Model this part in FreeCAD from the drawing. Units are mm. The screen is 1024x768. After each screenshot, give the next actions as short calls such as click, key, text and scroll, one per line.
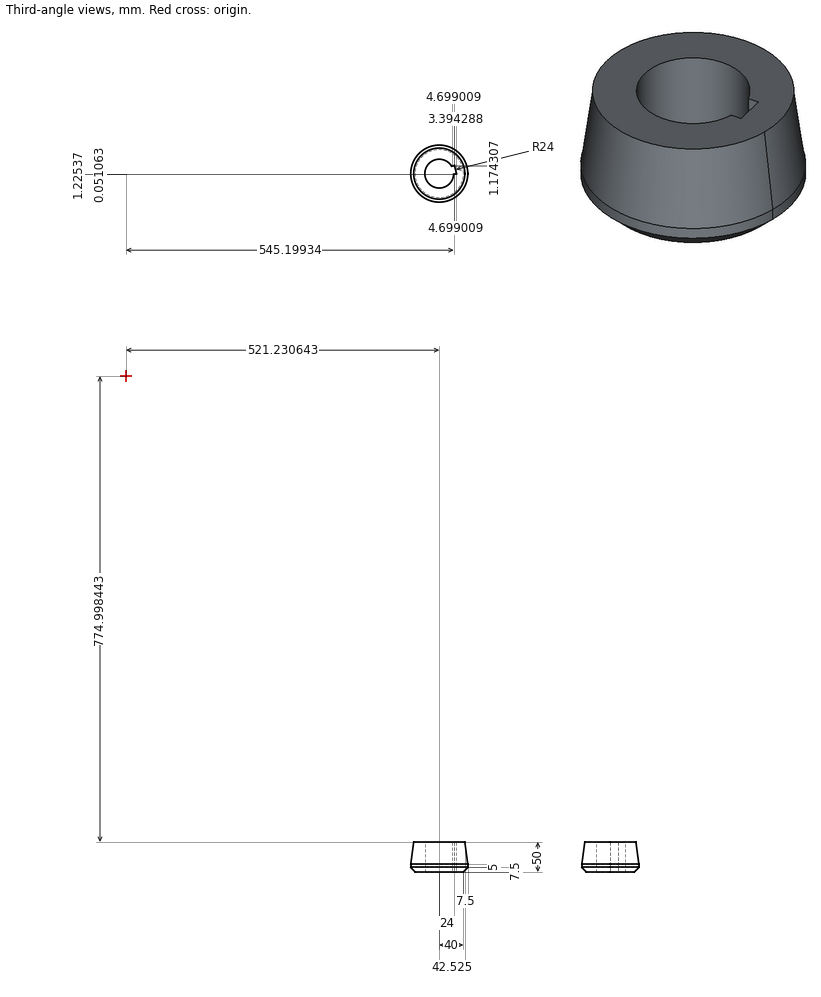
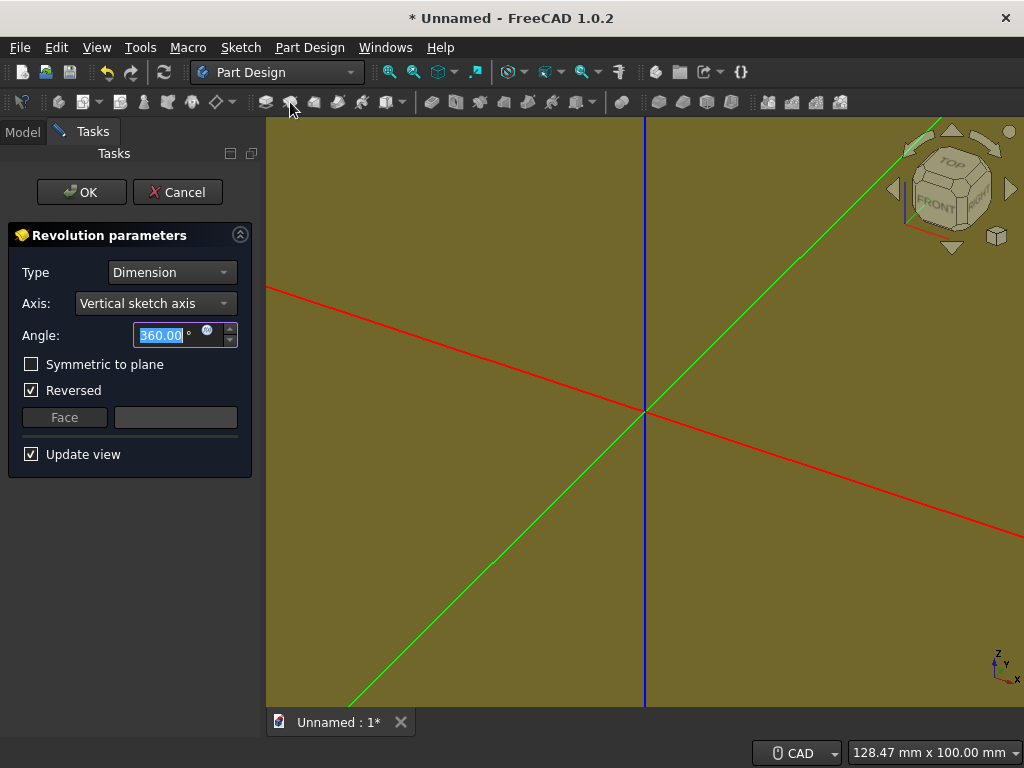
click(156, 304)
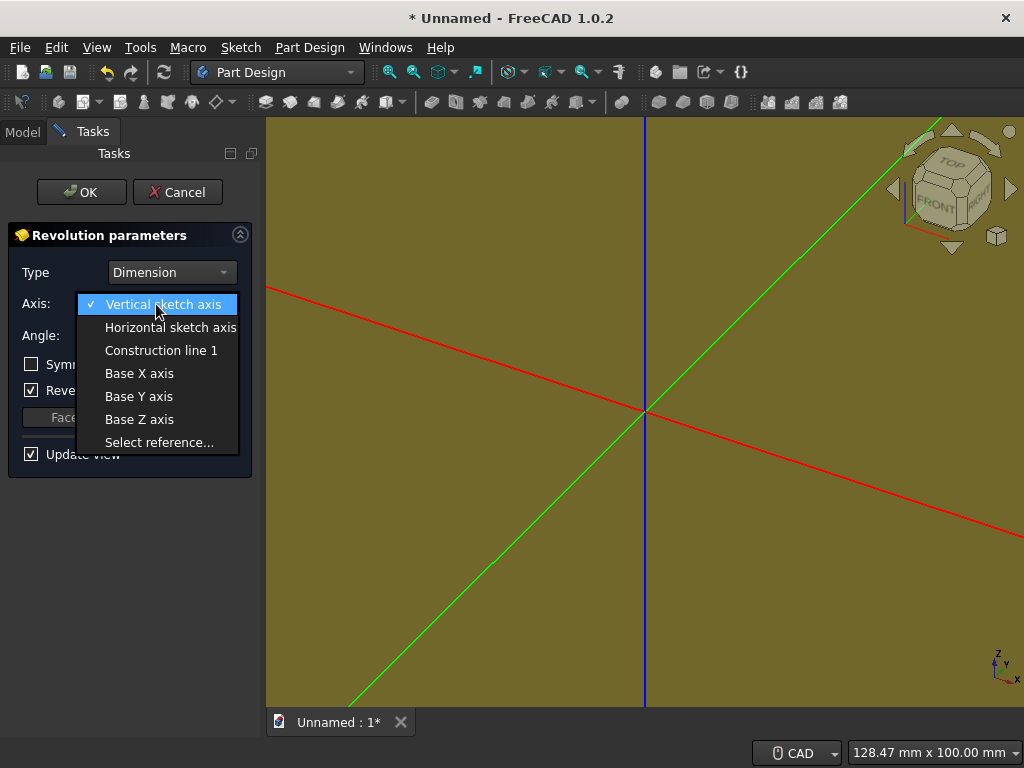
click(156, 350)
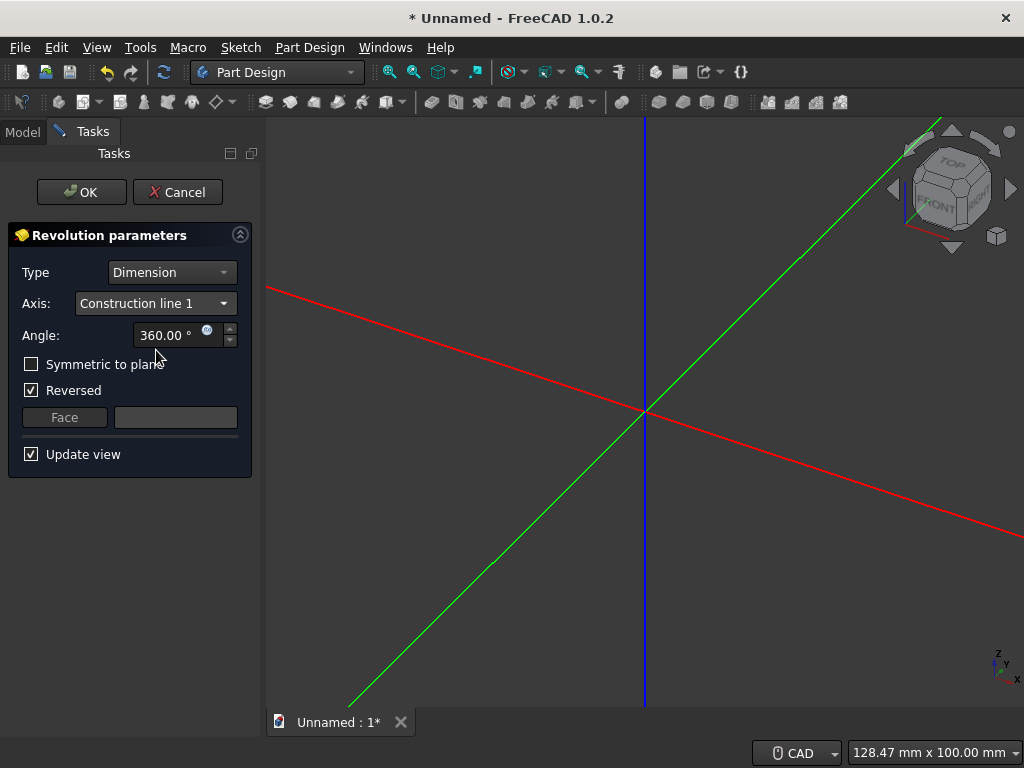
click(82, 192)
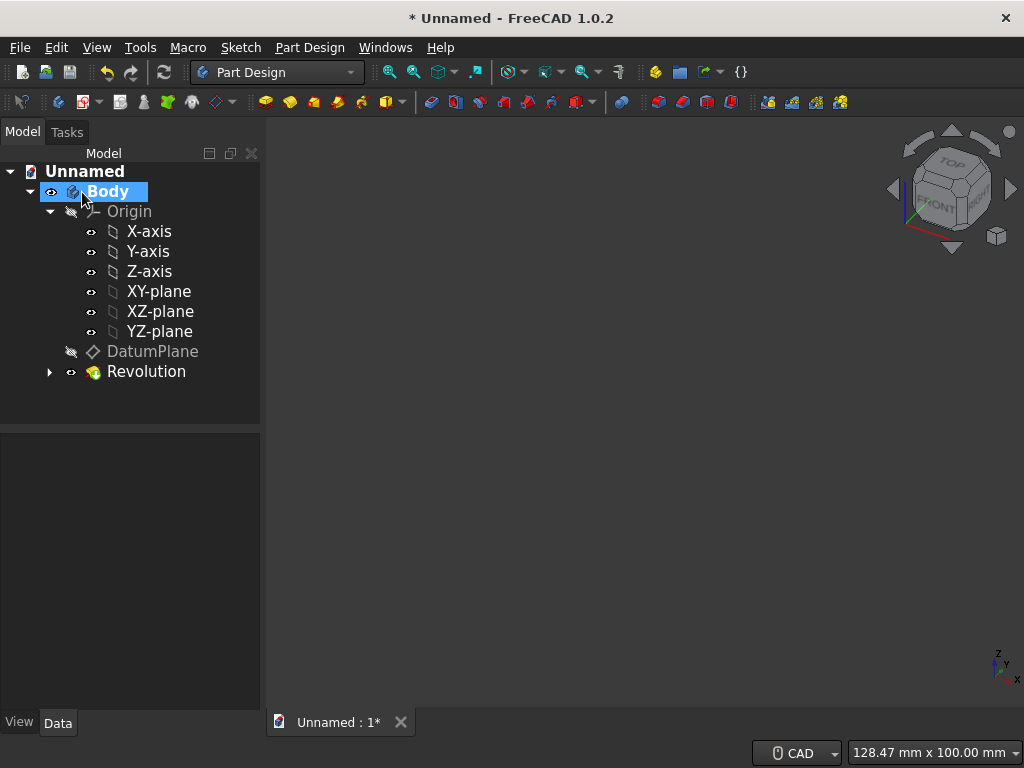
click(390, 72)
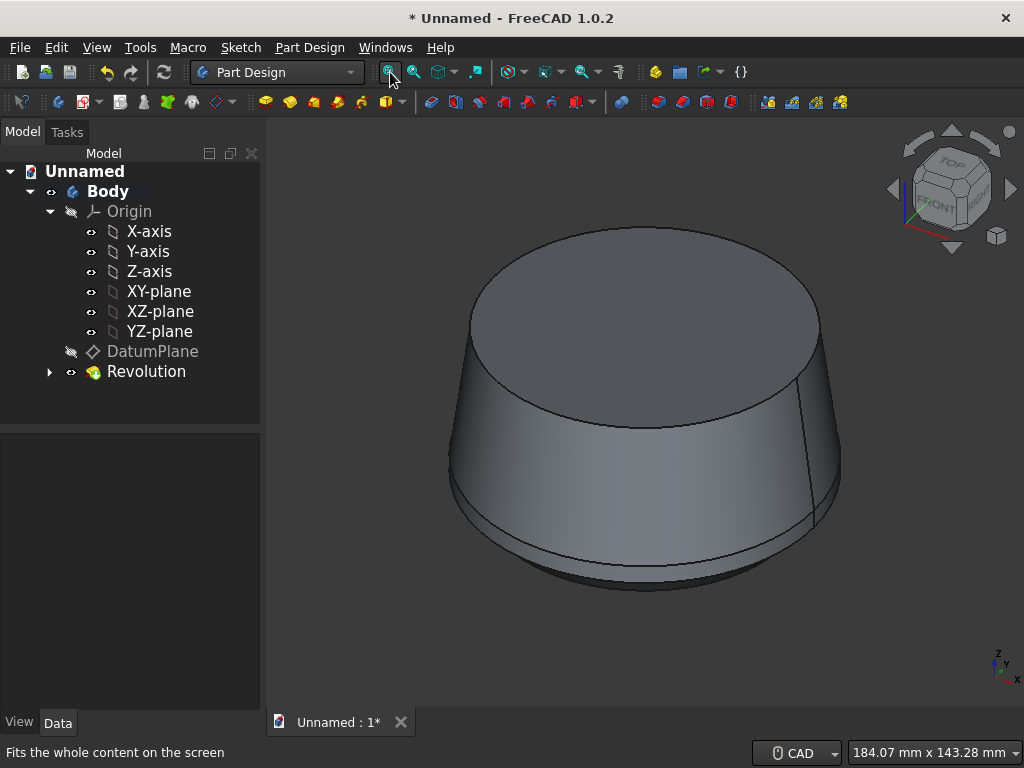
click(645, 327)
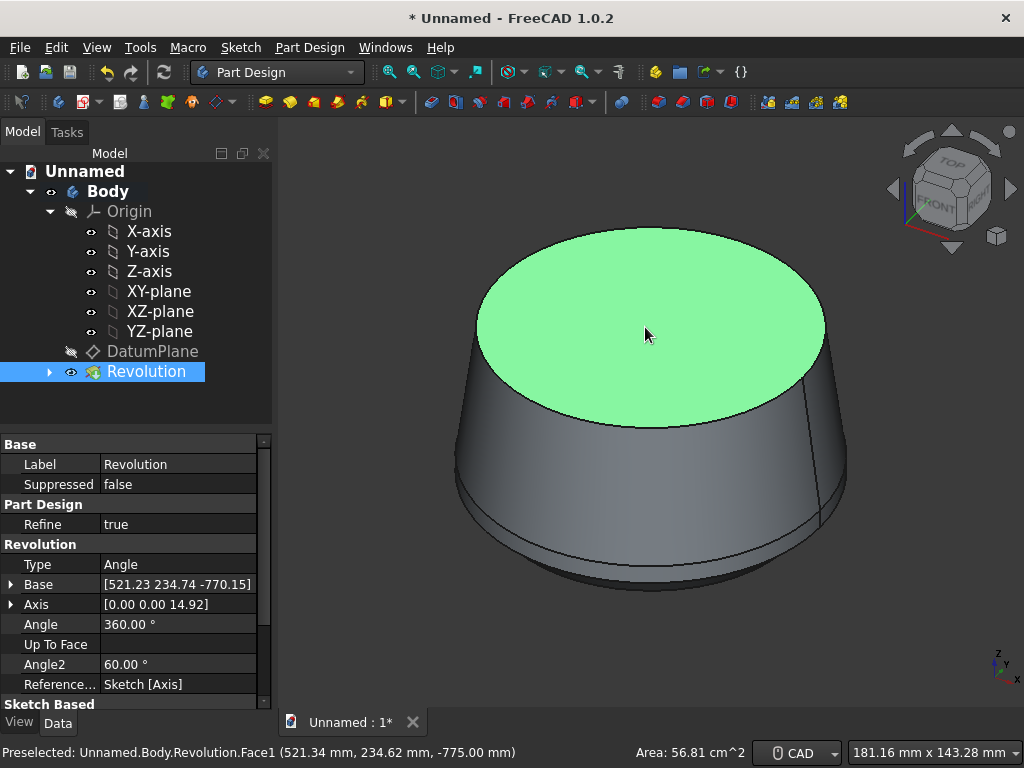
click(84, 102)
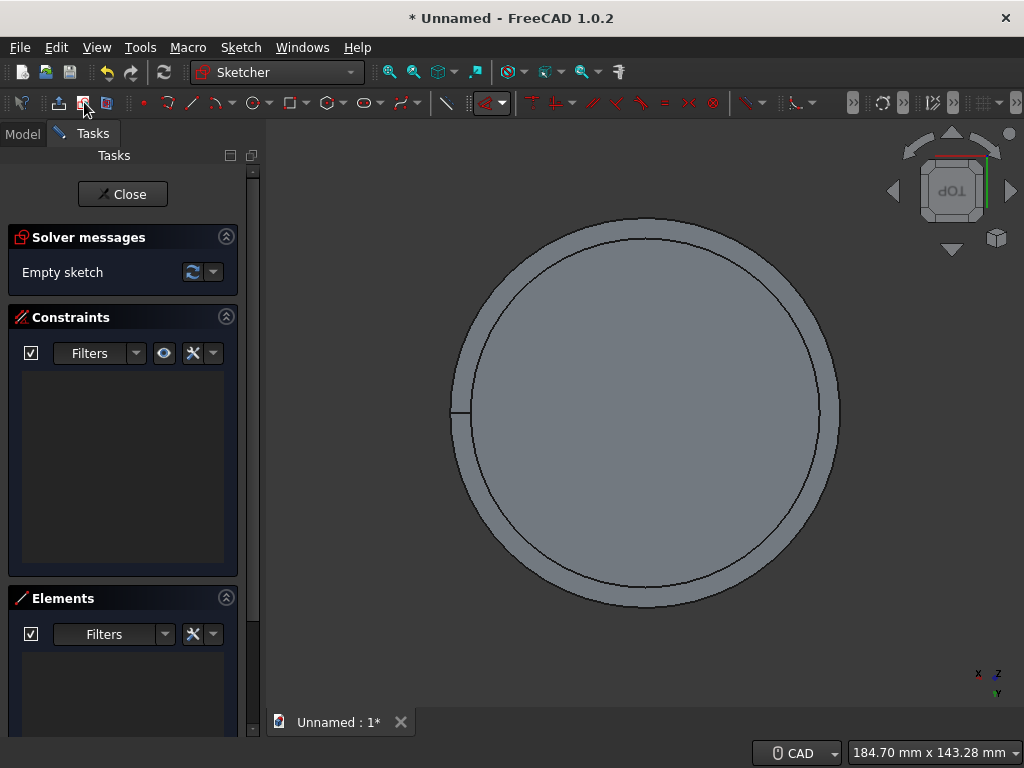
scroll(538, 443, up, 9)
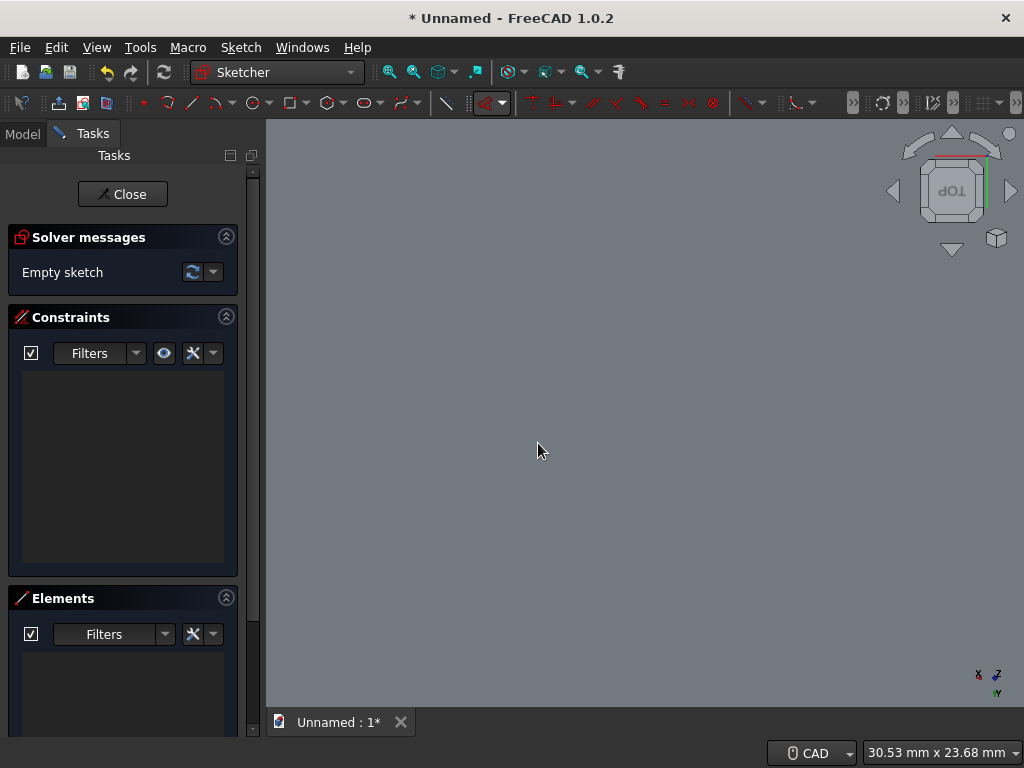
click(168, 104)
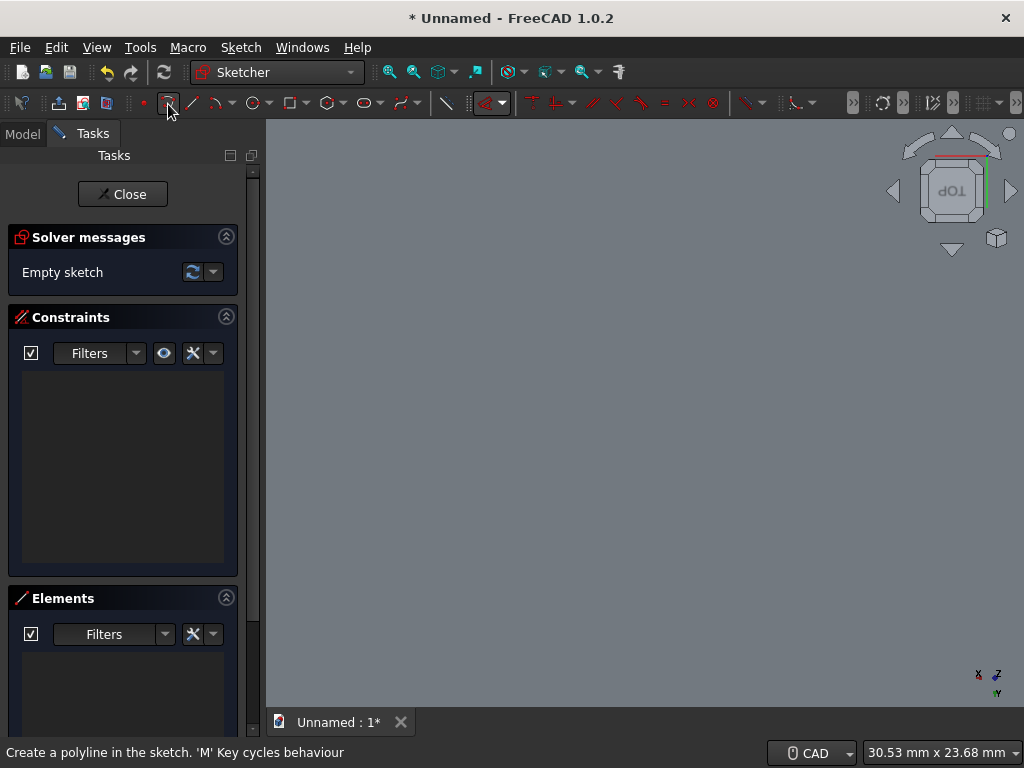
click(589, 228)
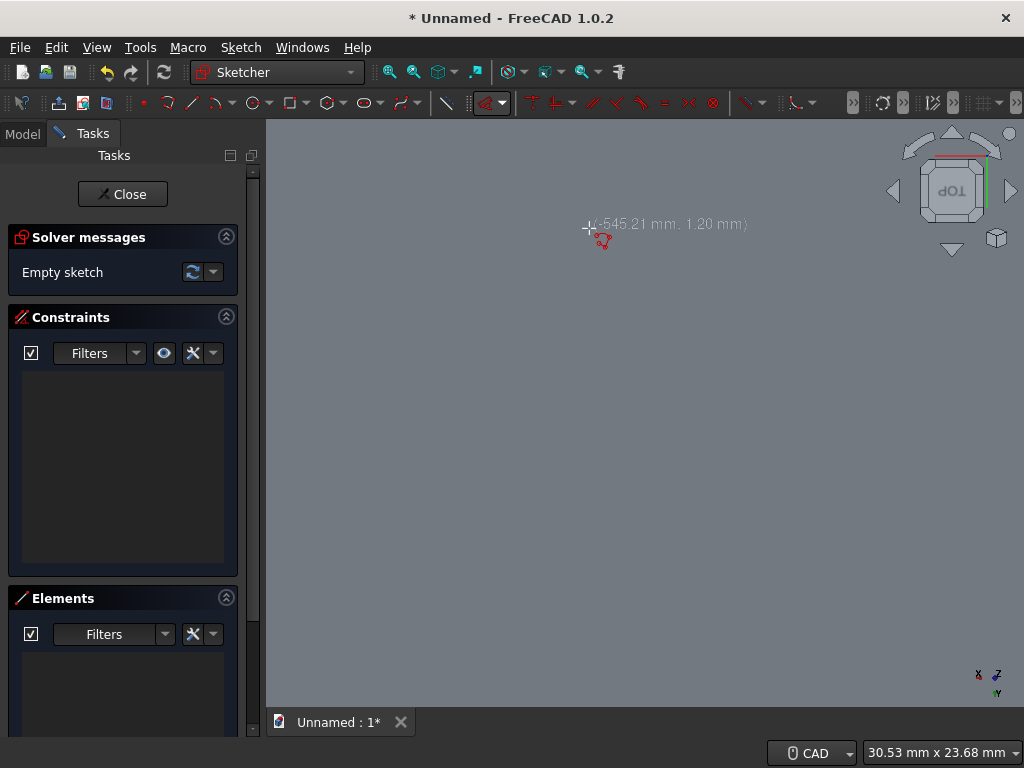
scroll(473, 257, up, 13)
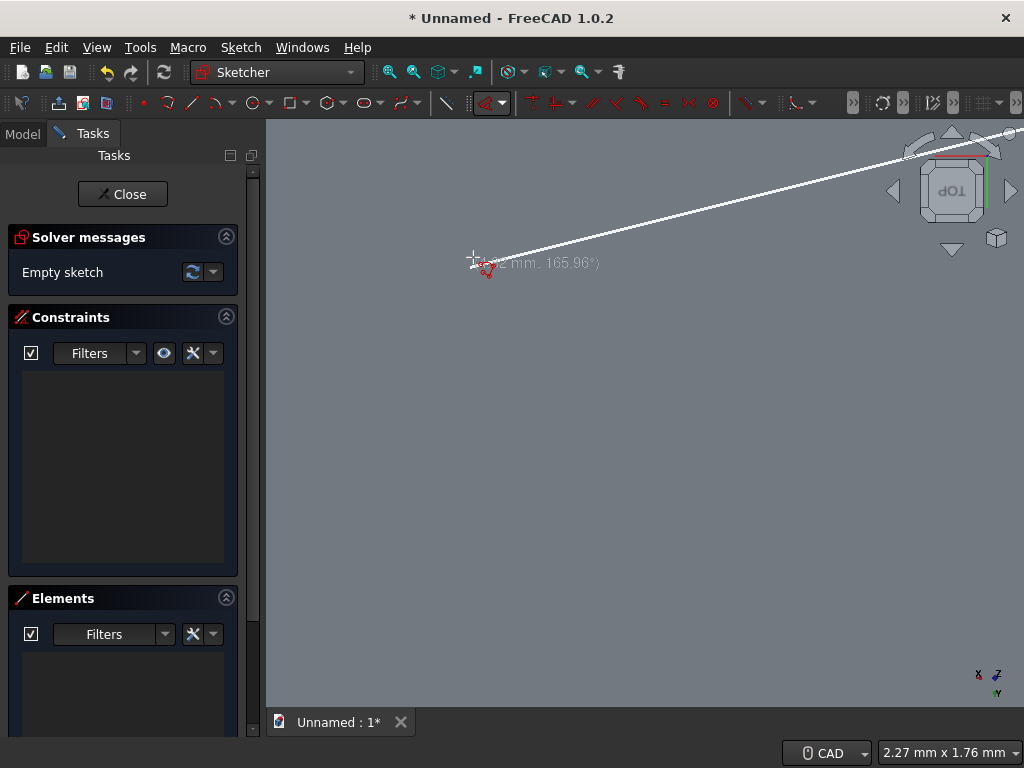
click(466, 260)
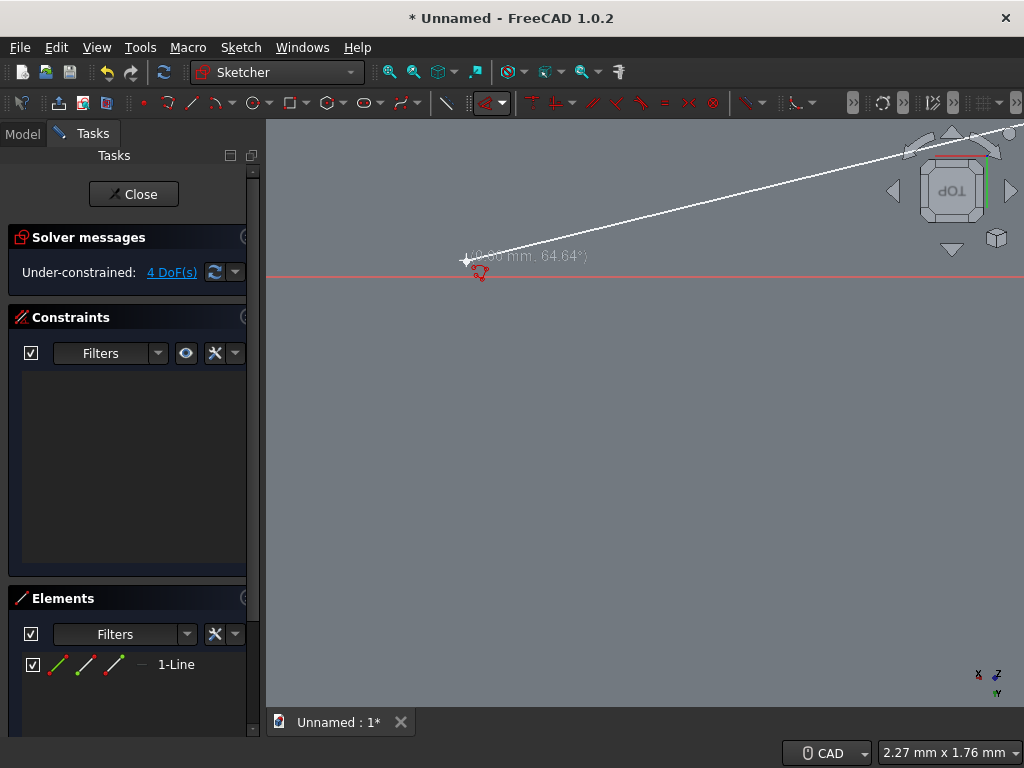
scroll(477, 259, down, 13)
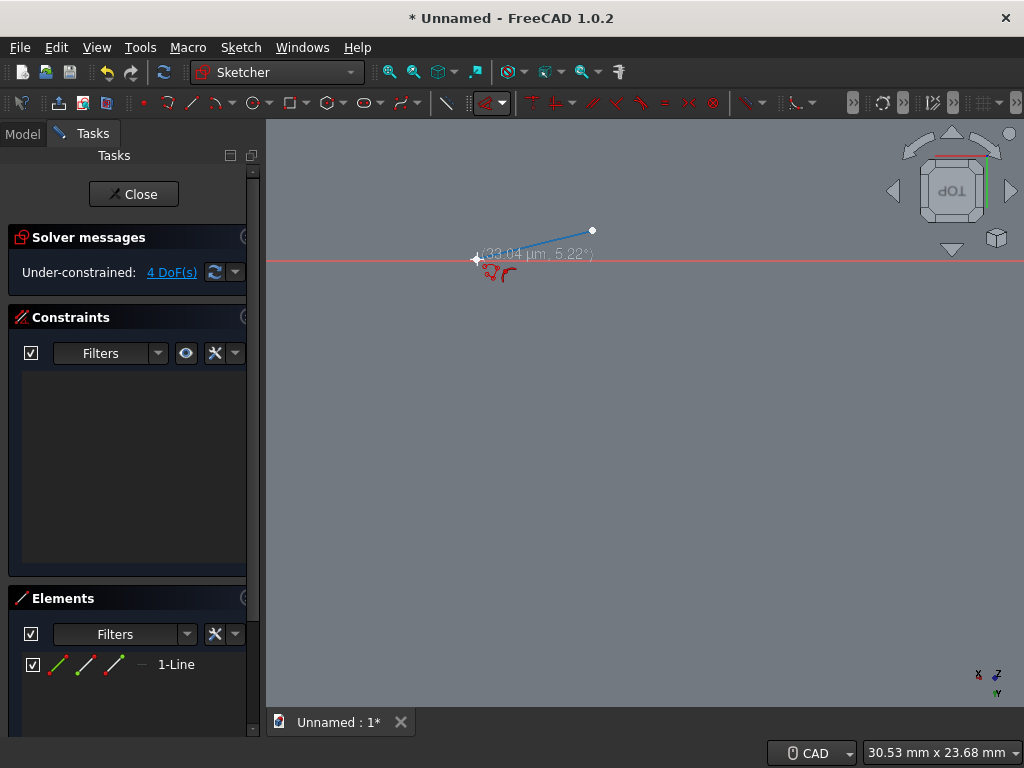
click(561, 597)
click(677, 567)
right_click(677, 567)